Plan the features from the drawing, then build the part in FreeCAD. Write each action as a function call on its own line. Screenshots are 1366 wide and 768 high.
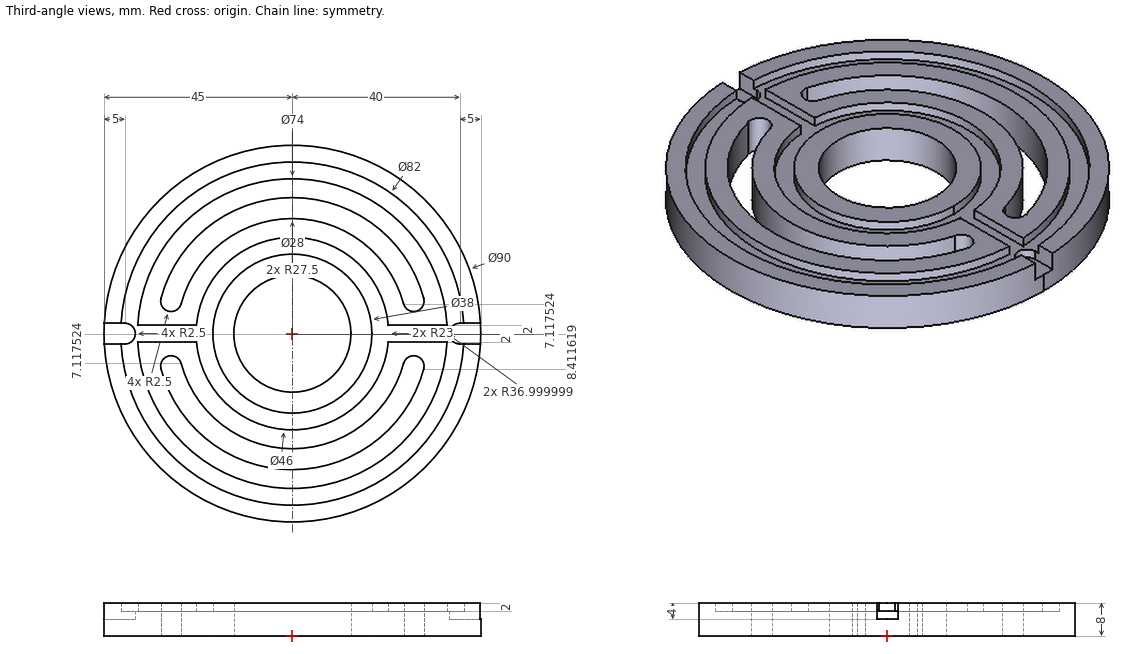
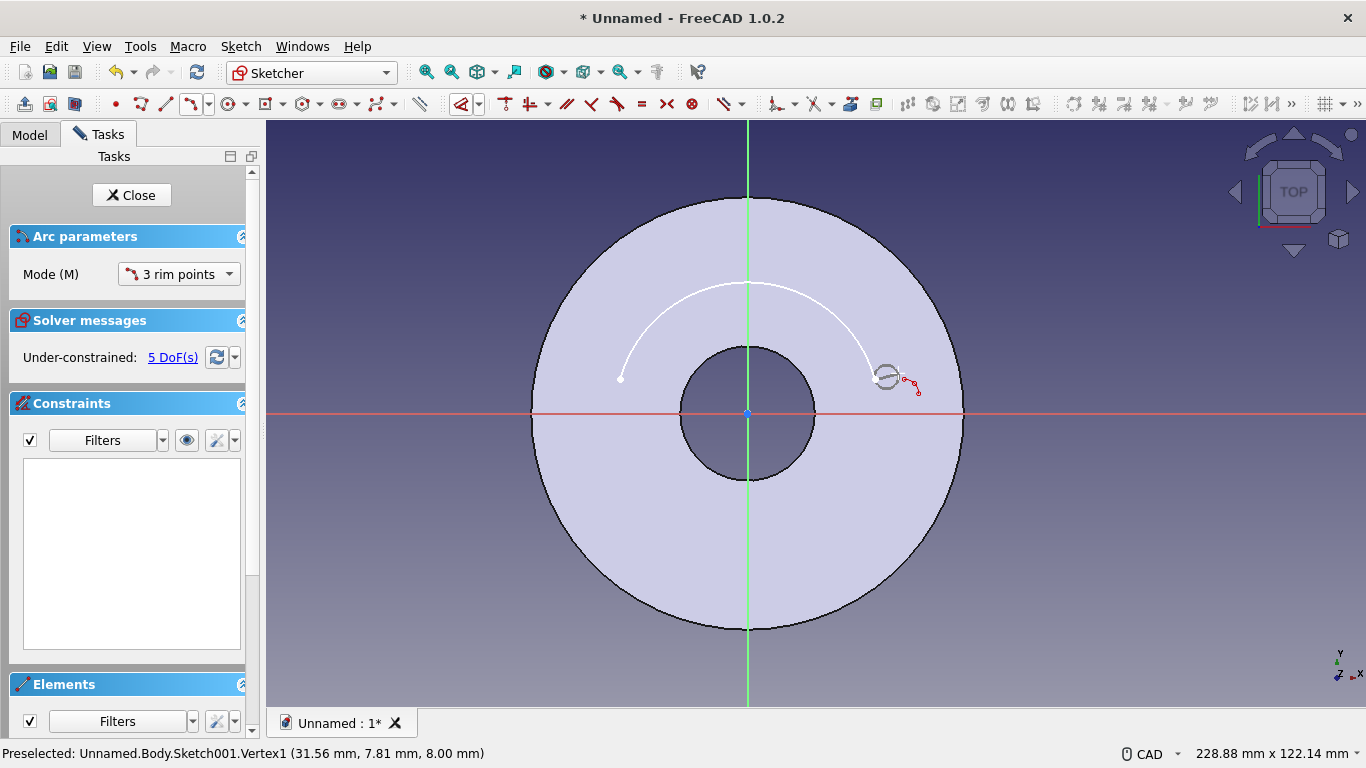
scroll(890, 388, up, 2)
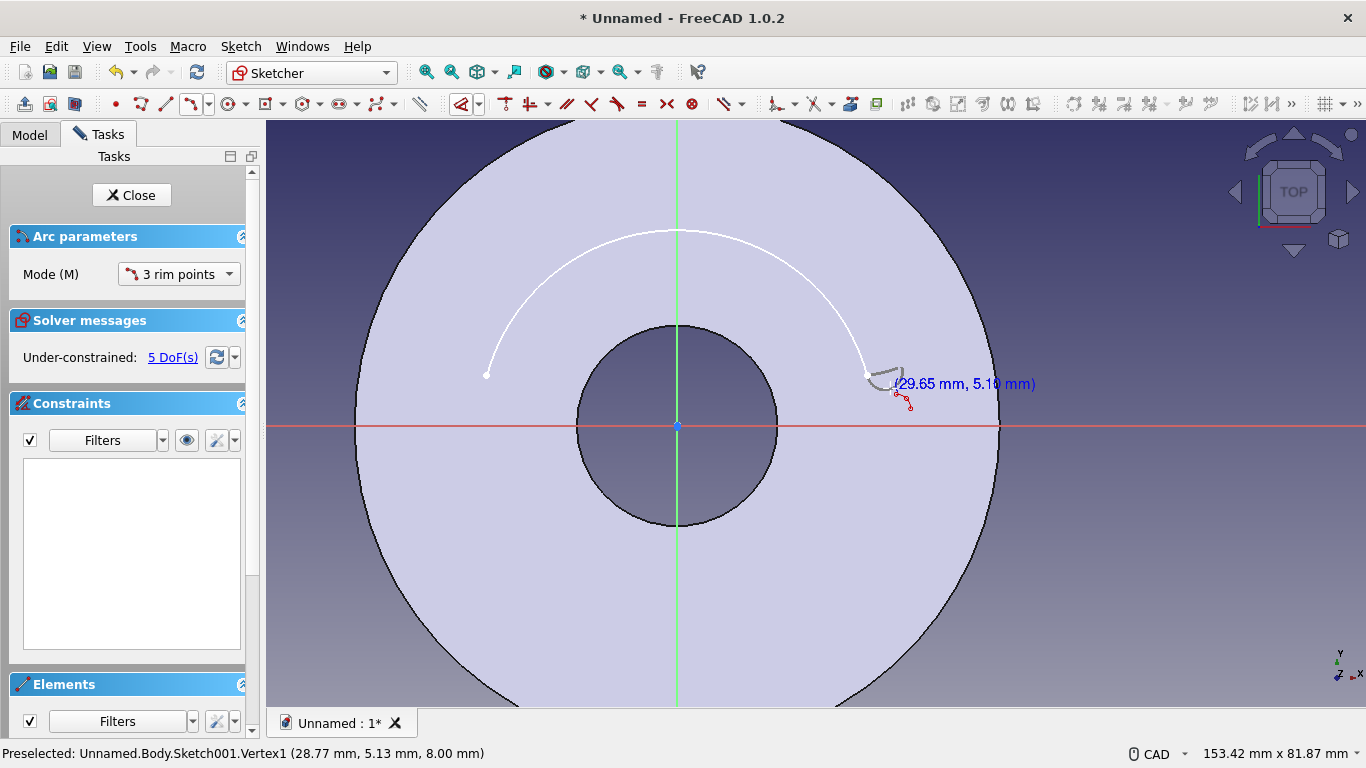
click(890, 387)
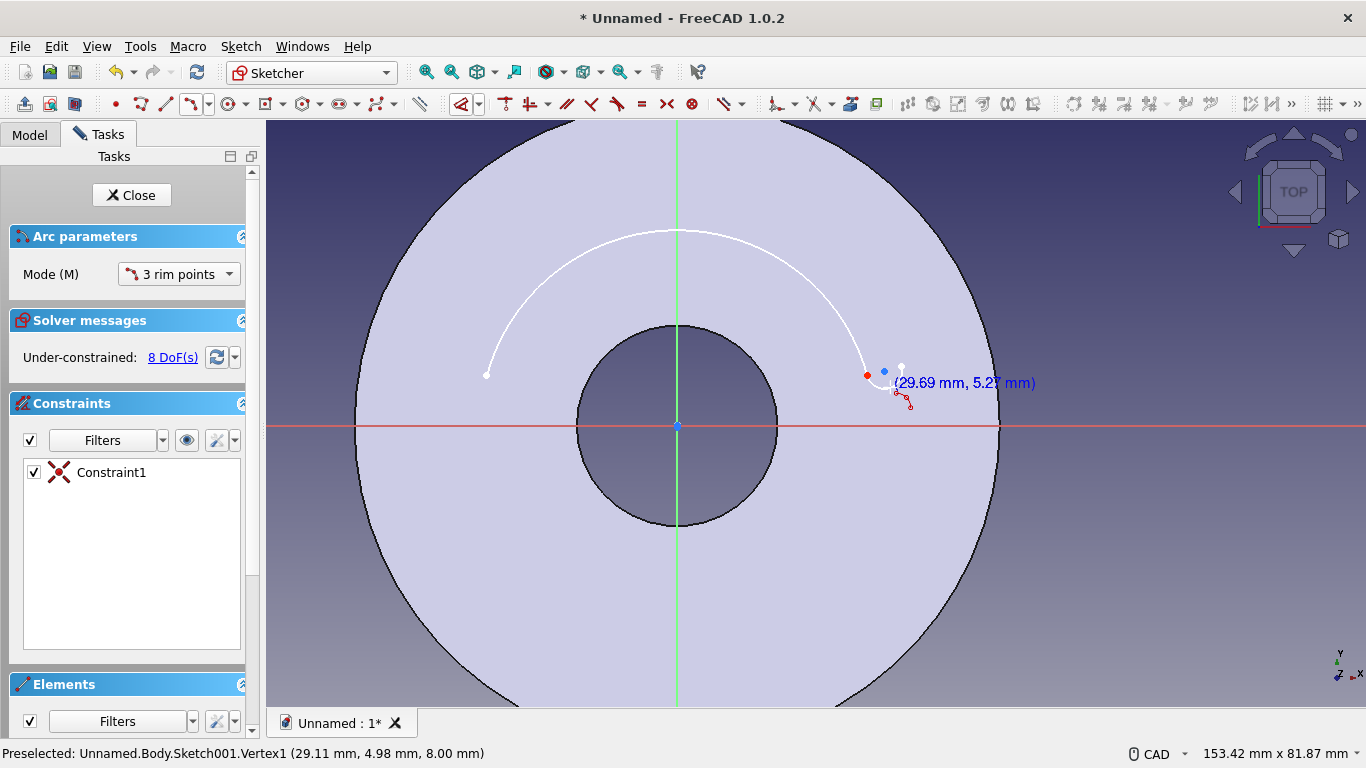
click(902, 367)
click(452, 366)
click(737, 201)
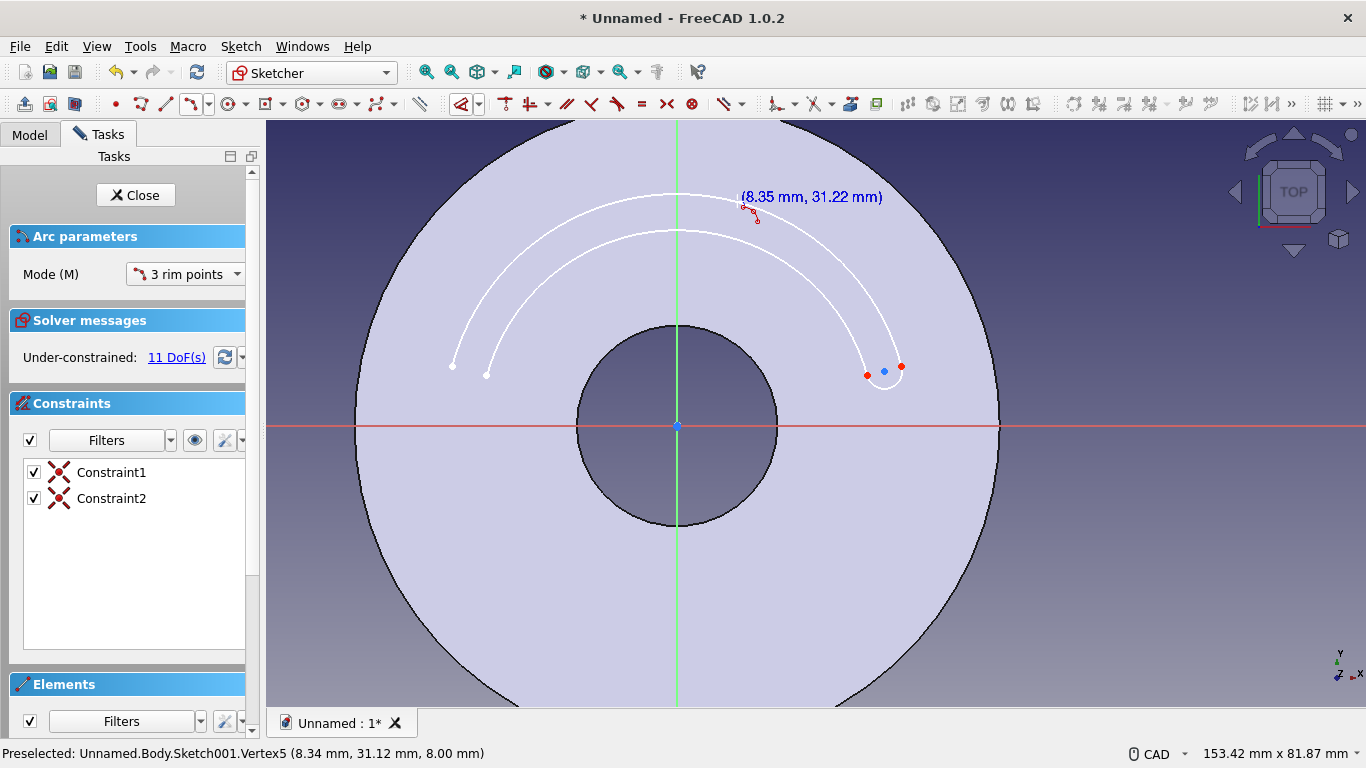
click(452, 367)
click(487, 376)
click(465, 387)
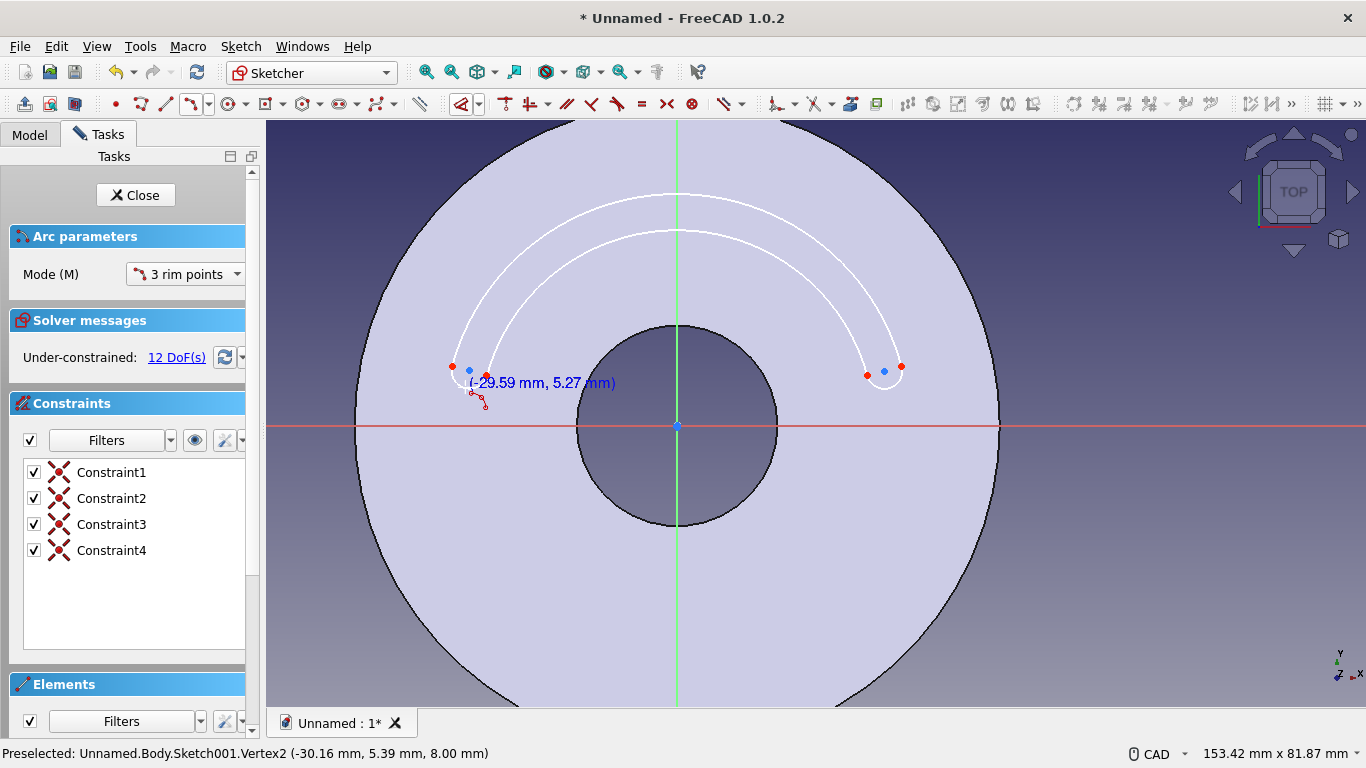
click(487, 477)
click(452, 486)
click(465, 464)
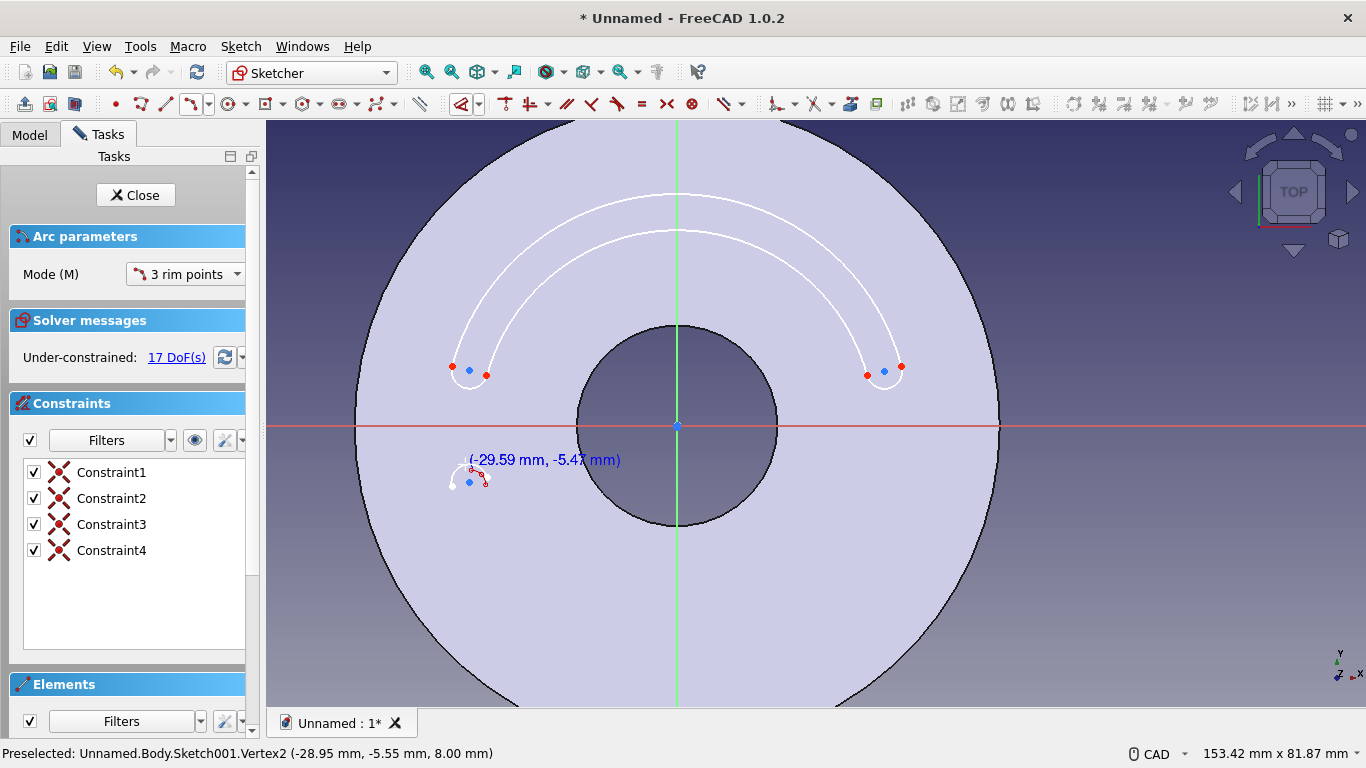
click(452, 487)
click(902, 486)
click(617, 651)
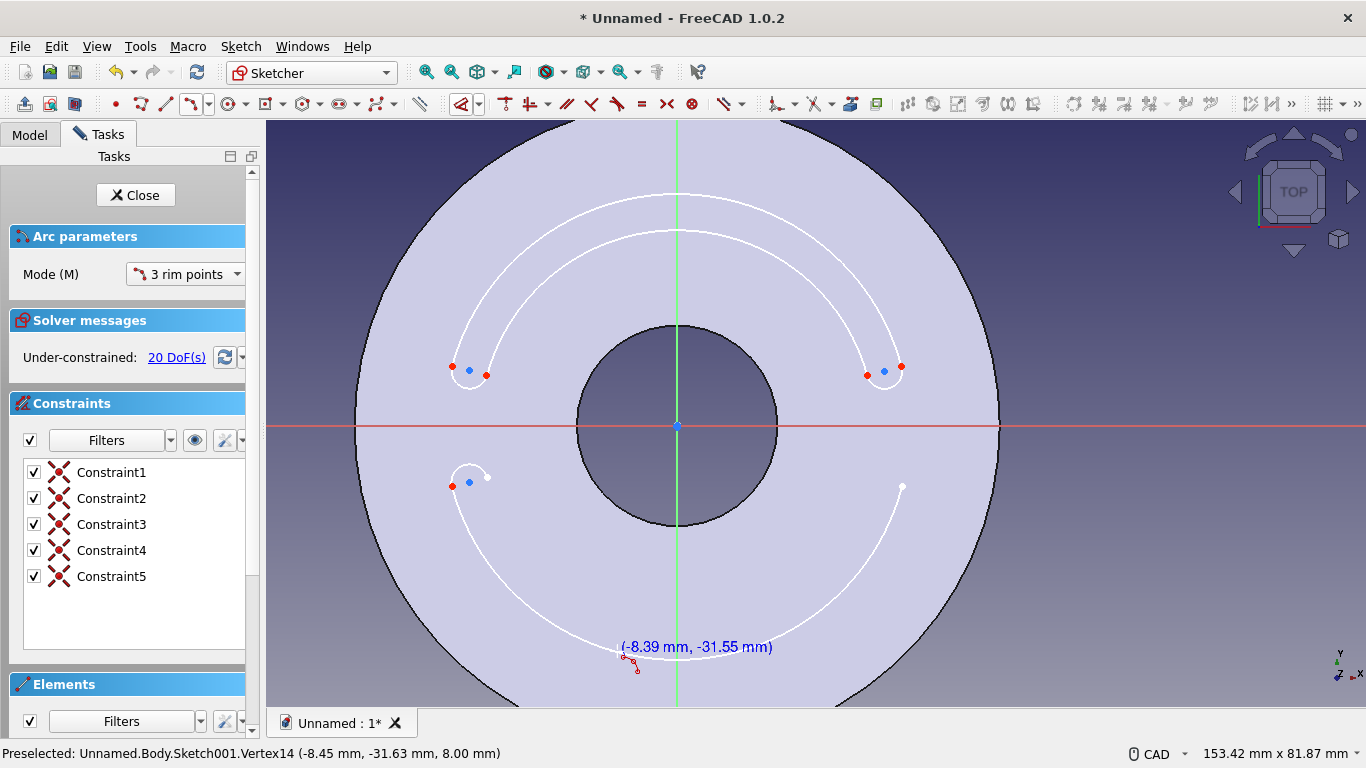
click(902, 487)
click(868, 477)
click(890, 464)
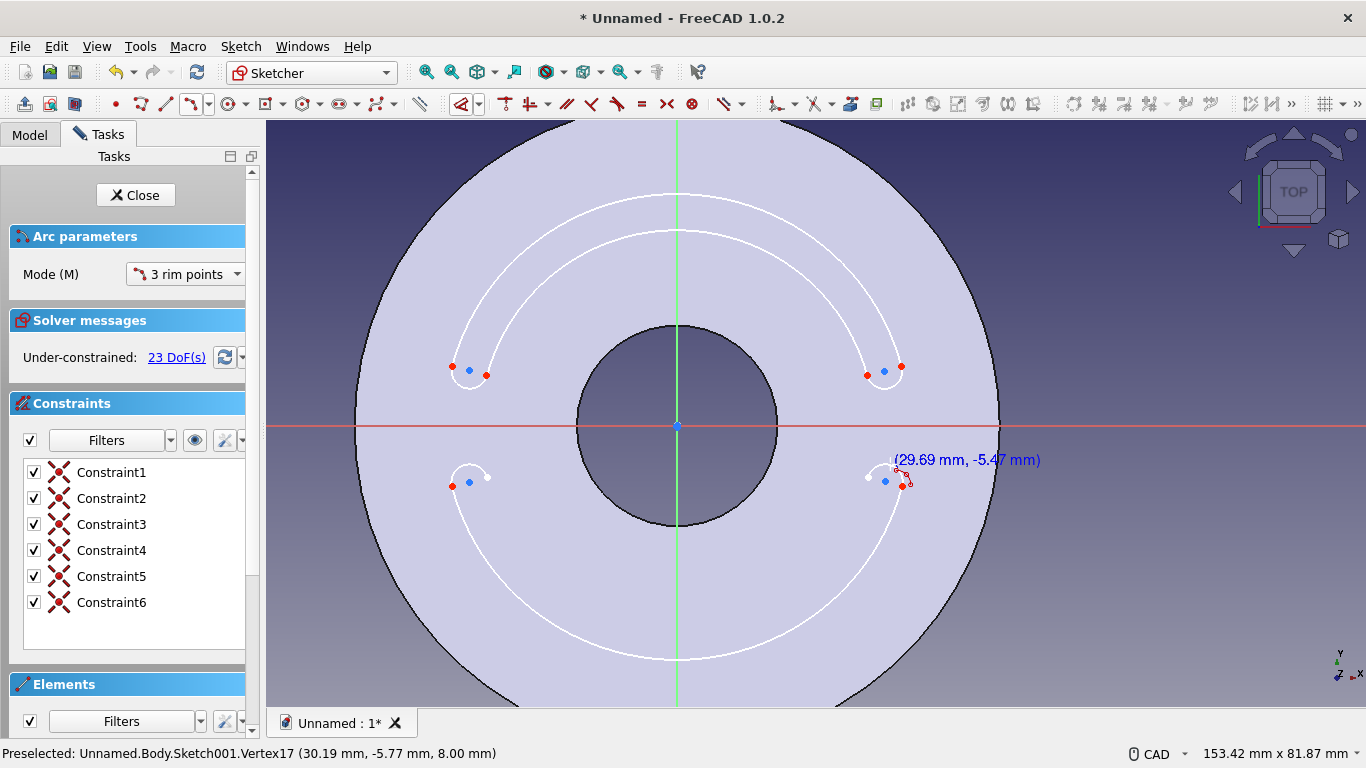
click(868, 478)
click(487, 478)
click(626, 616)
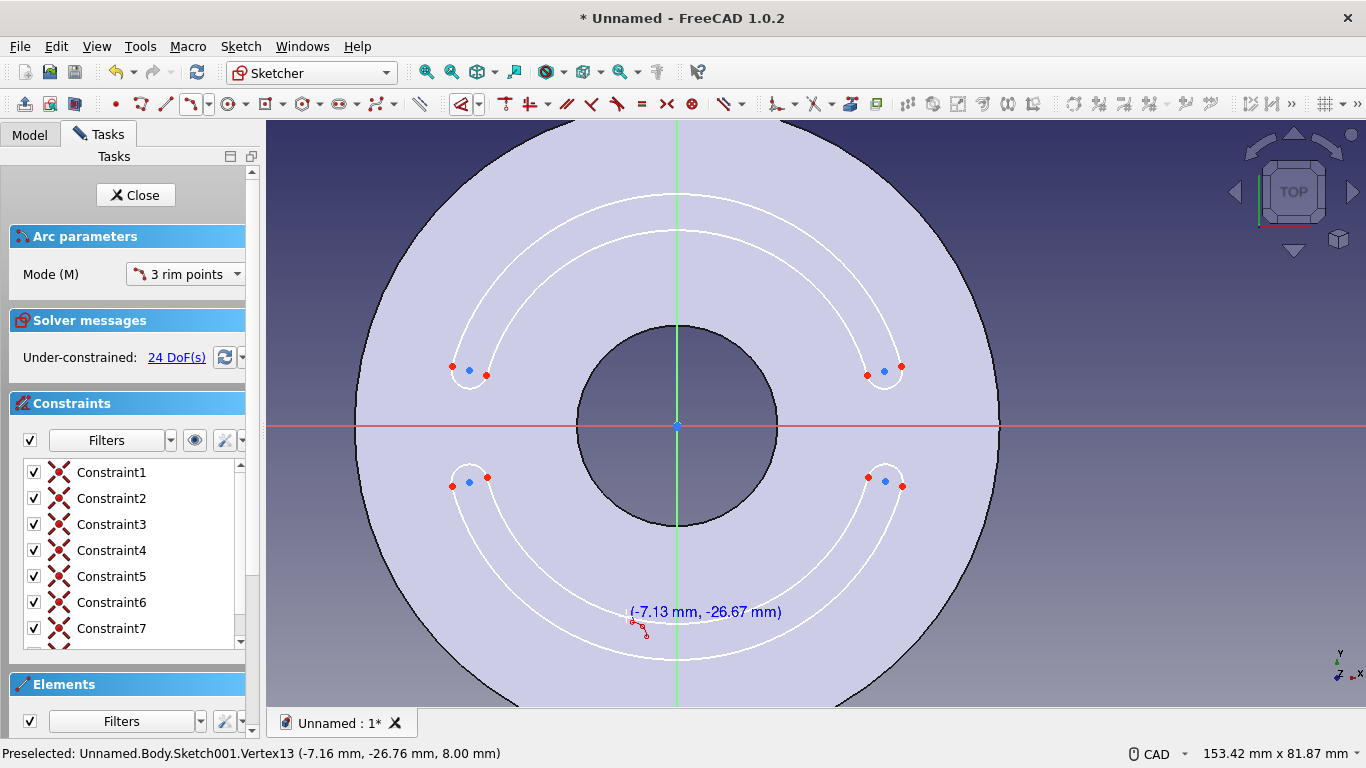
key(g)
key(c)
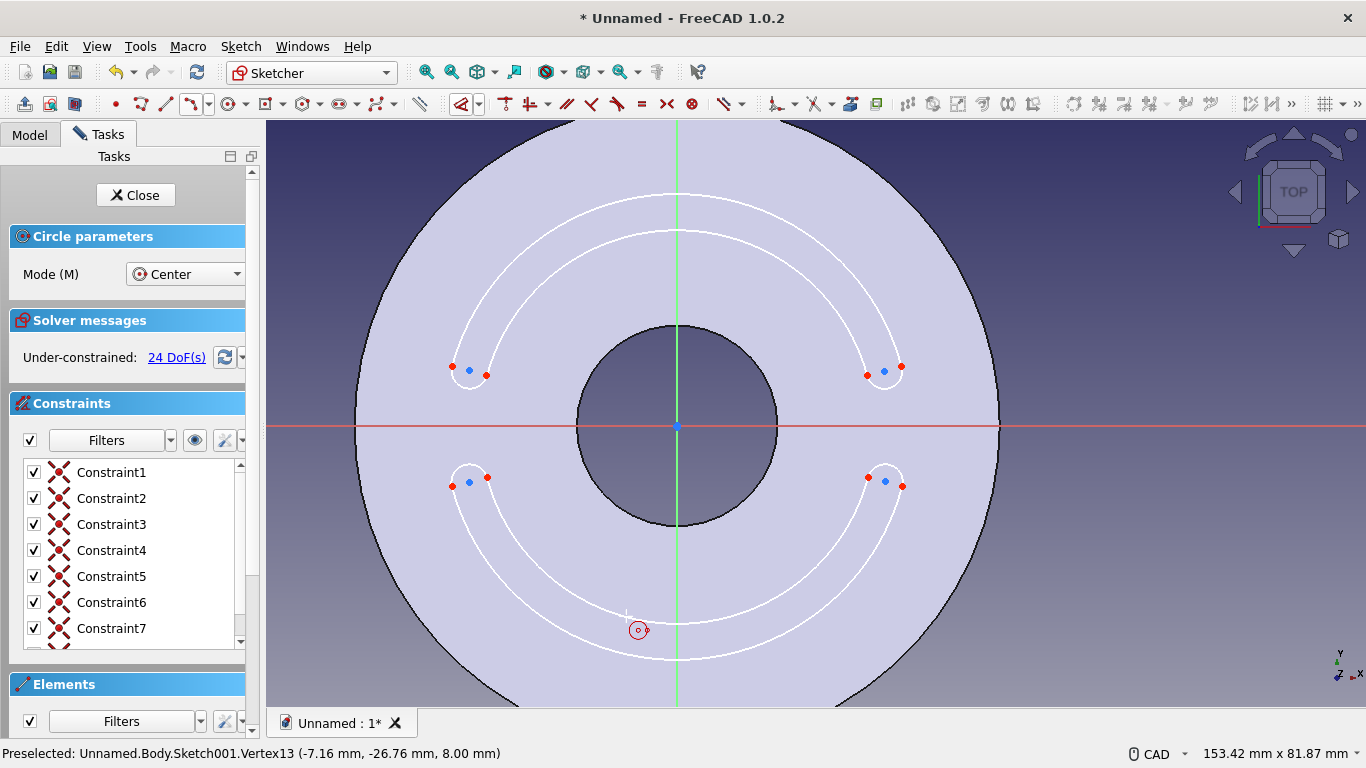
click(677, 426)
move(885, 218)